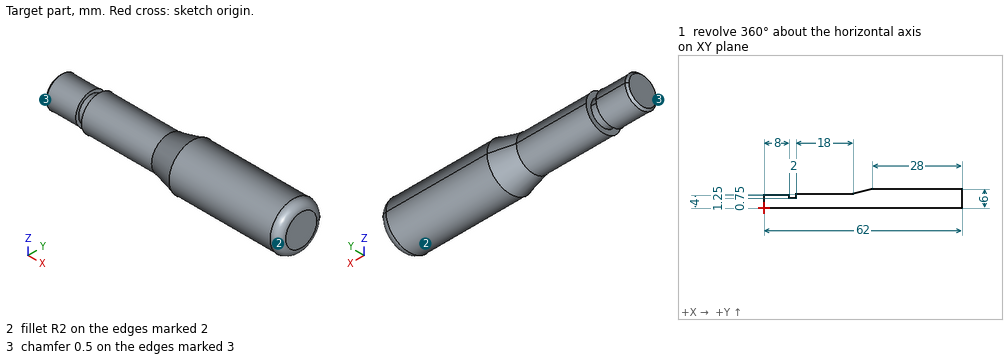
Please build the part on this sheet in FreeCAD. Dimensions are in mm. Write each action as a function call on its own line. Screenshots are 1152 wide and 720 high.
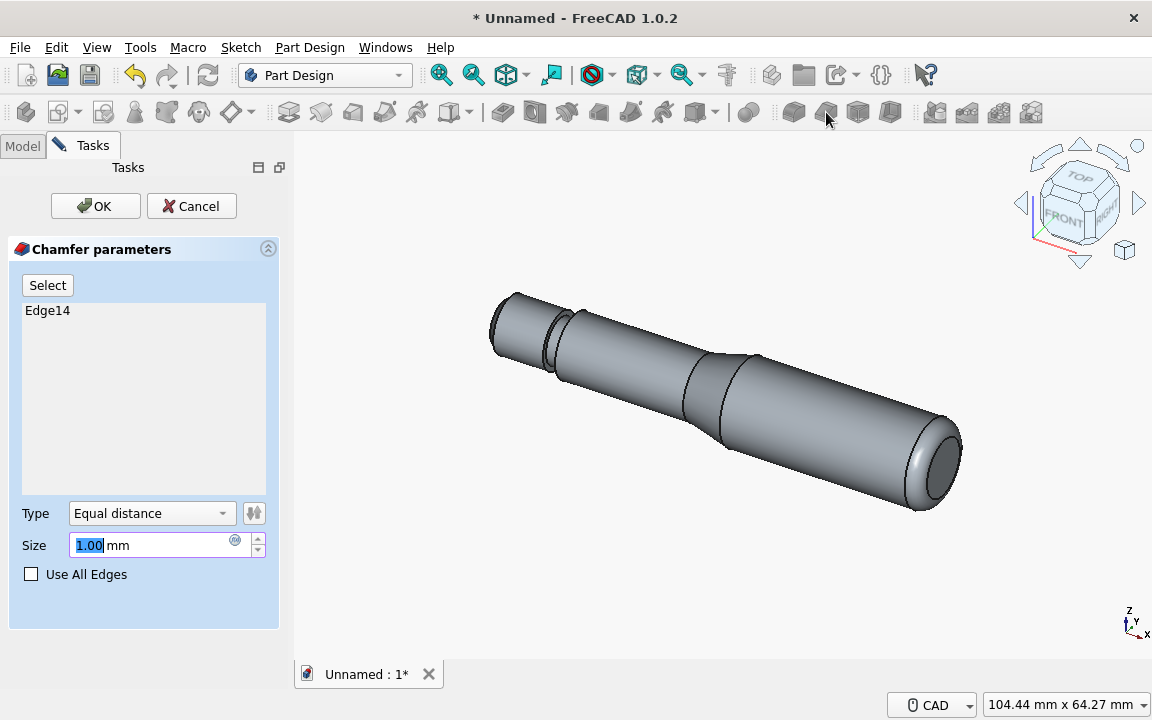
text(0.5)
key(Tab)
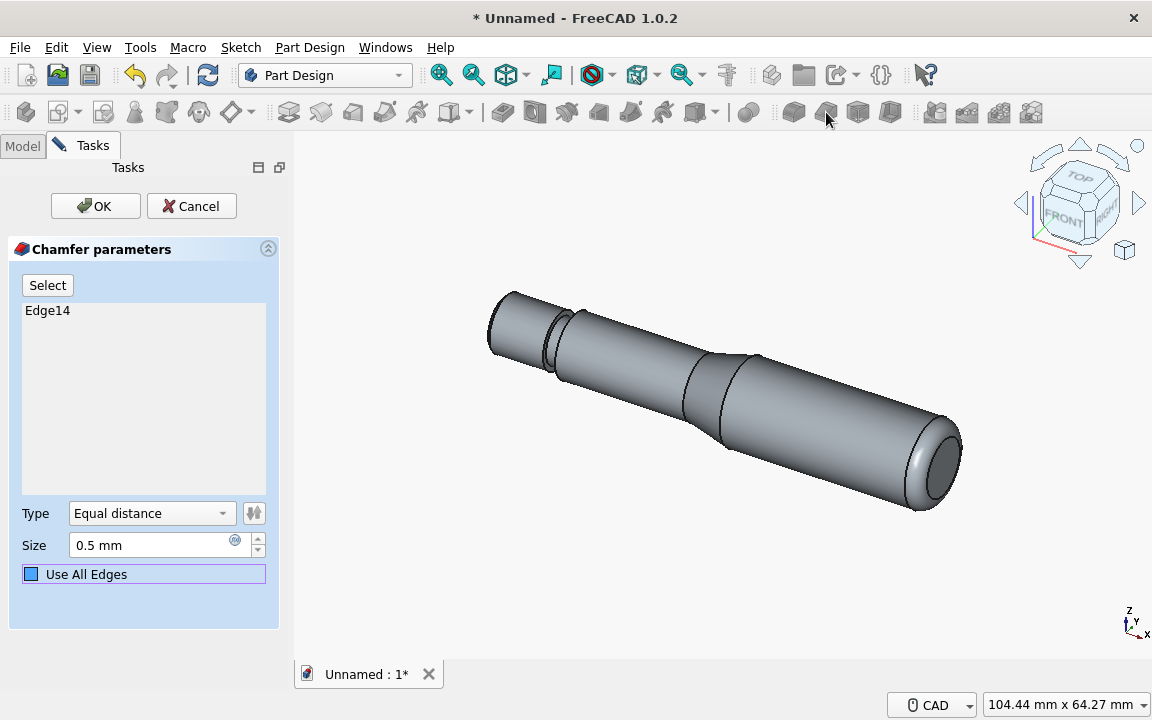
click(96, 206)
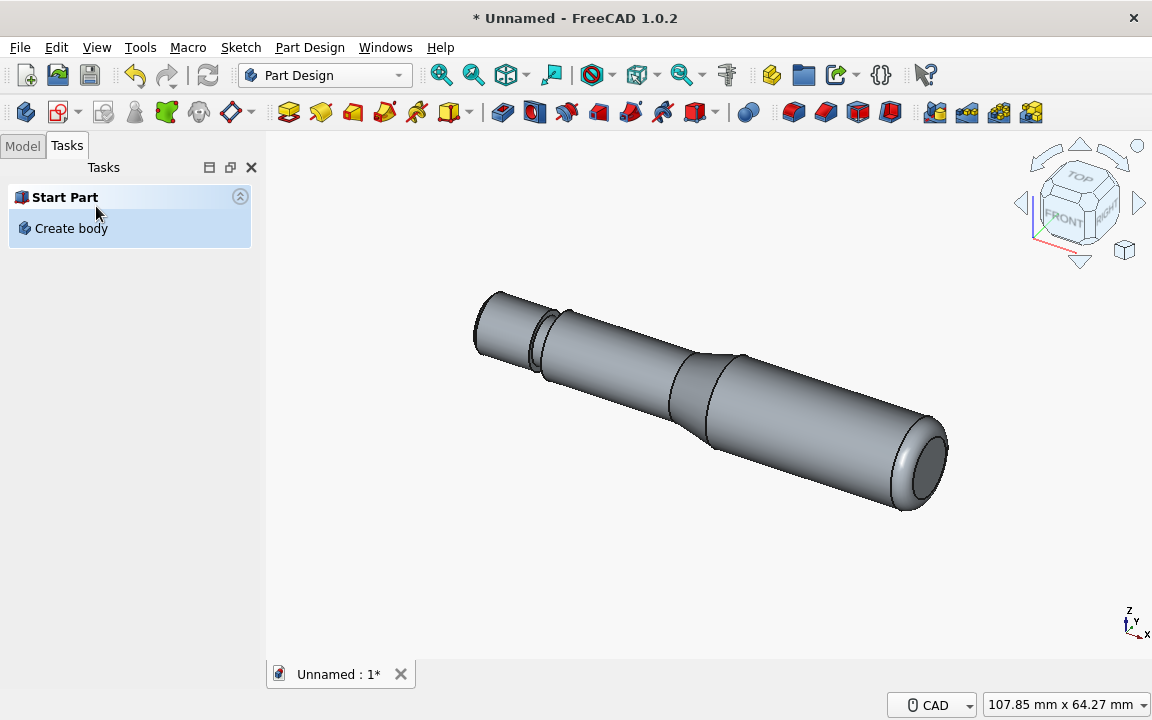
key(0)